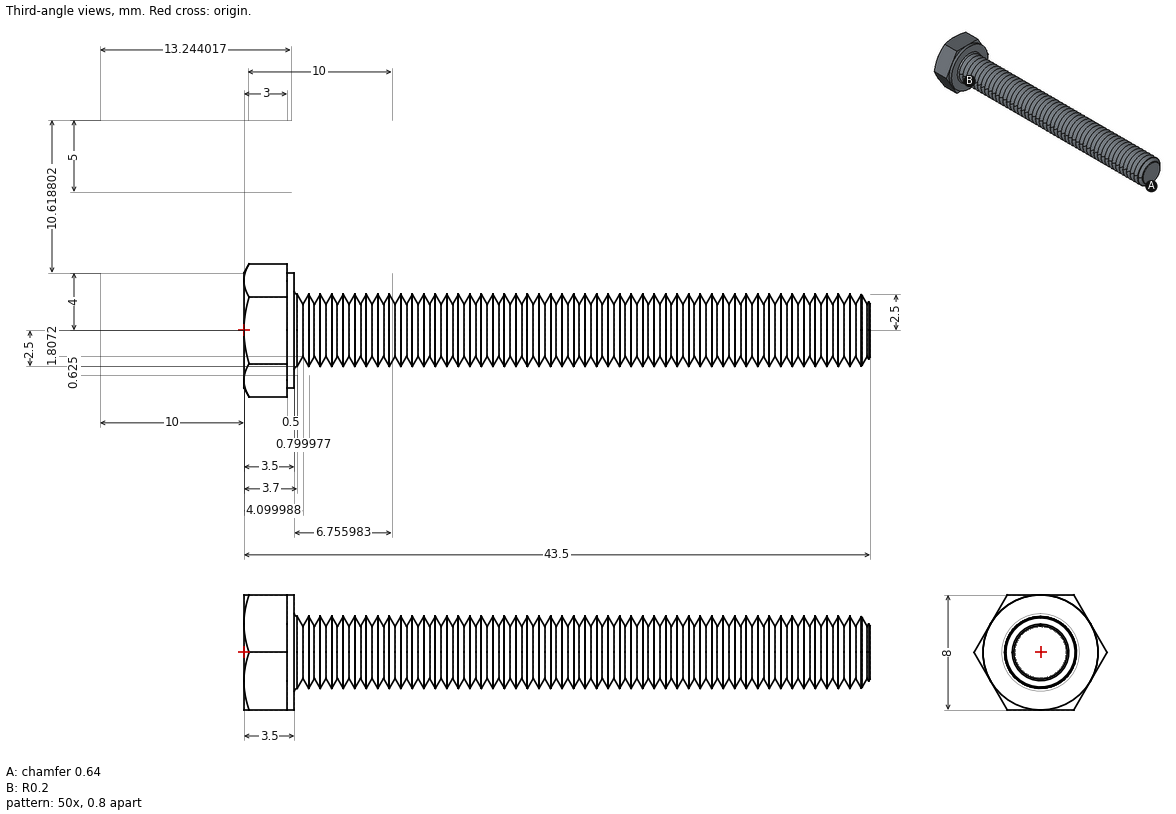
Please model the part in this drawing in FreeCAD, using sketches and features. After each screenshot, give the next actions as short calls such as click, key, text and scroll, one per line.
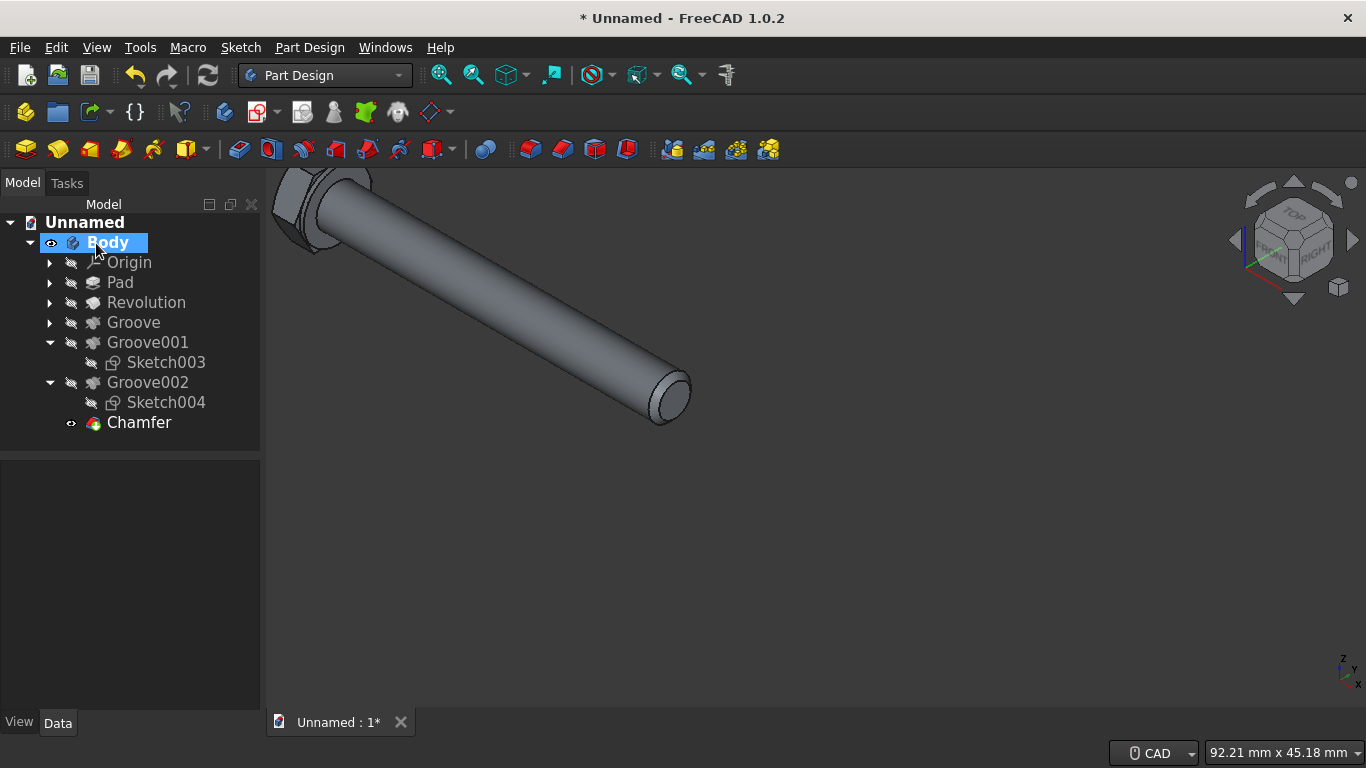
click(442, 76)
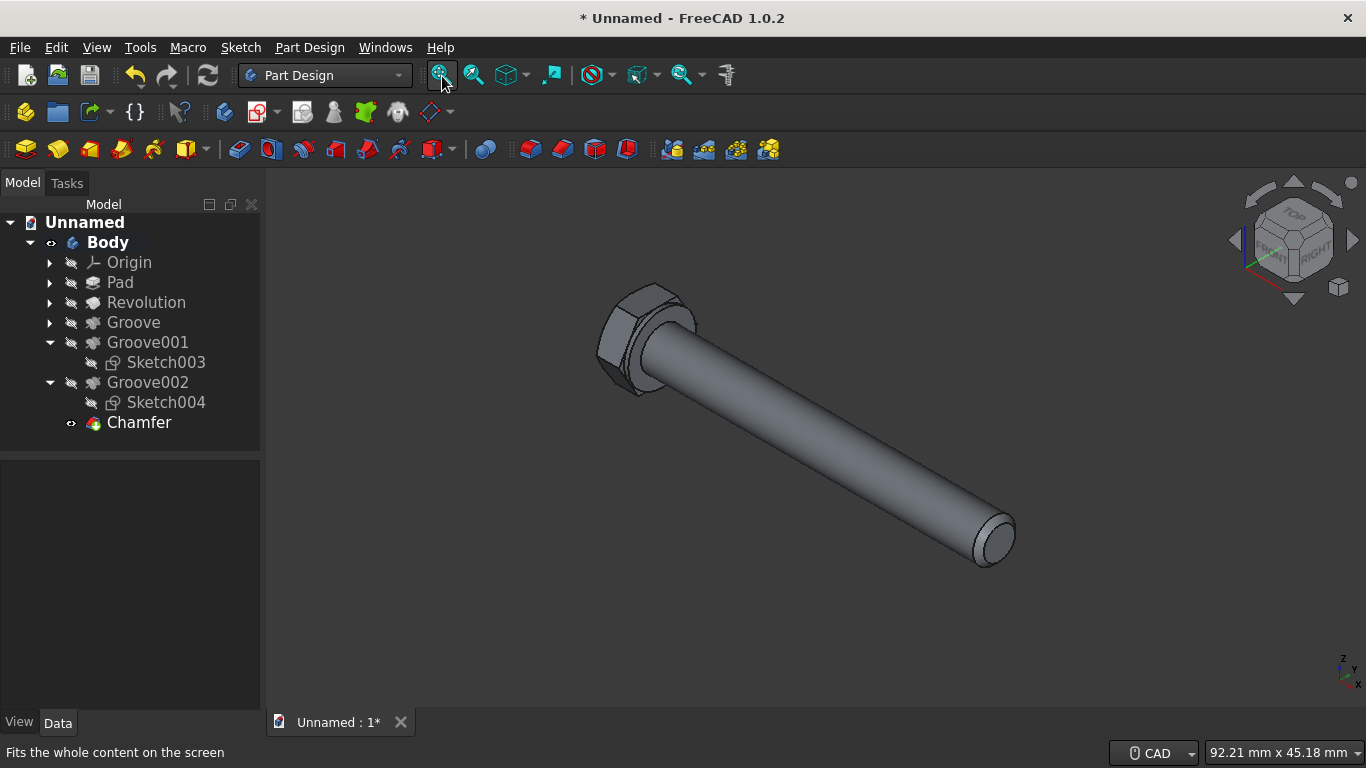
key(2)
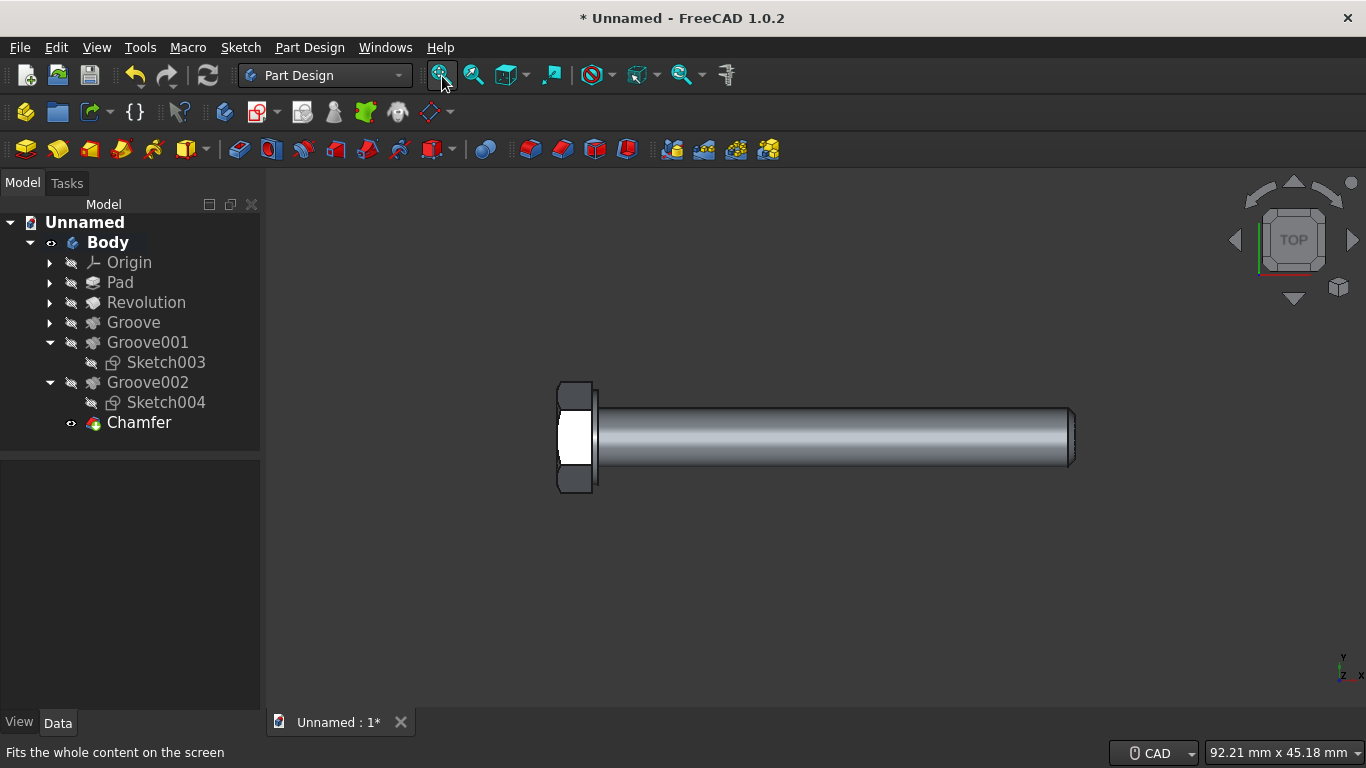
key(1)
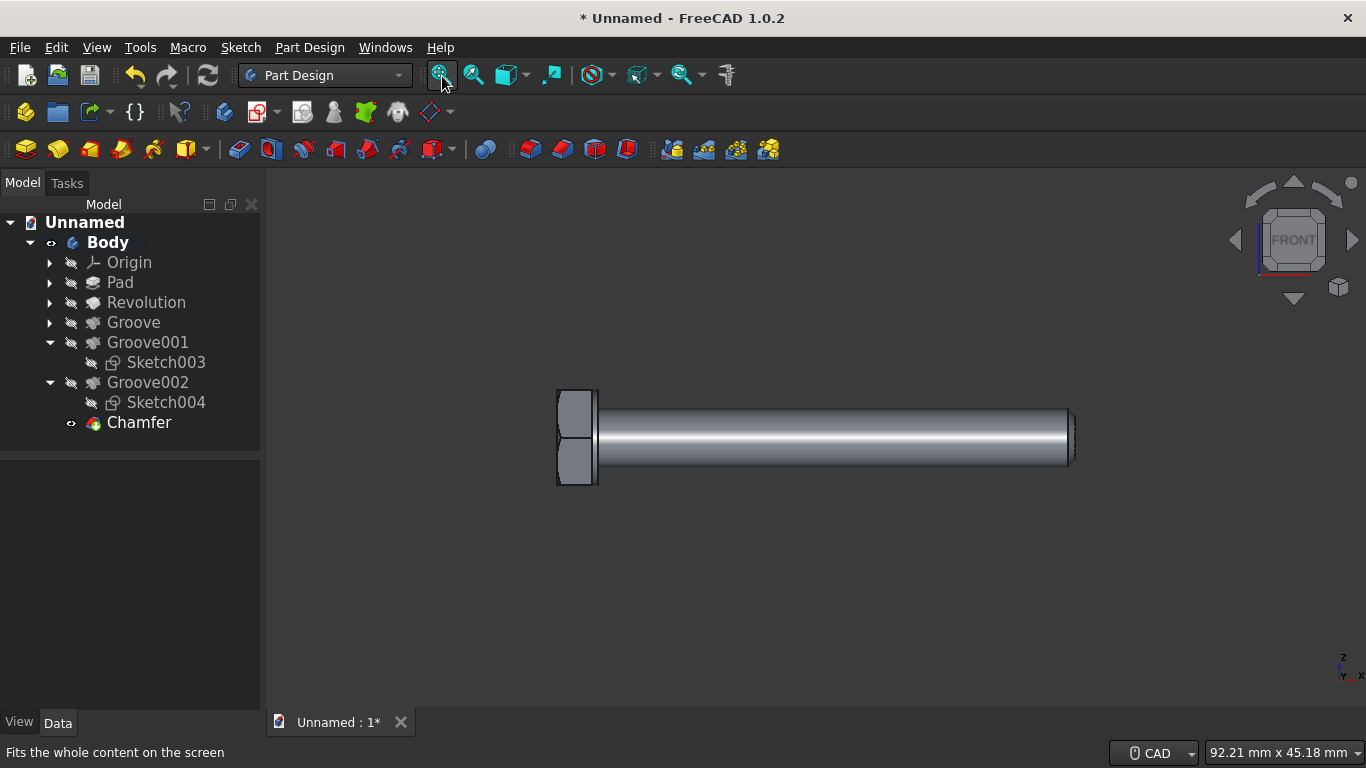
key(3)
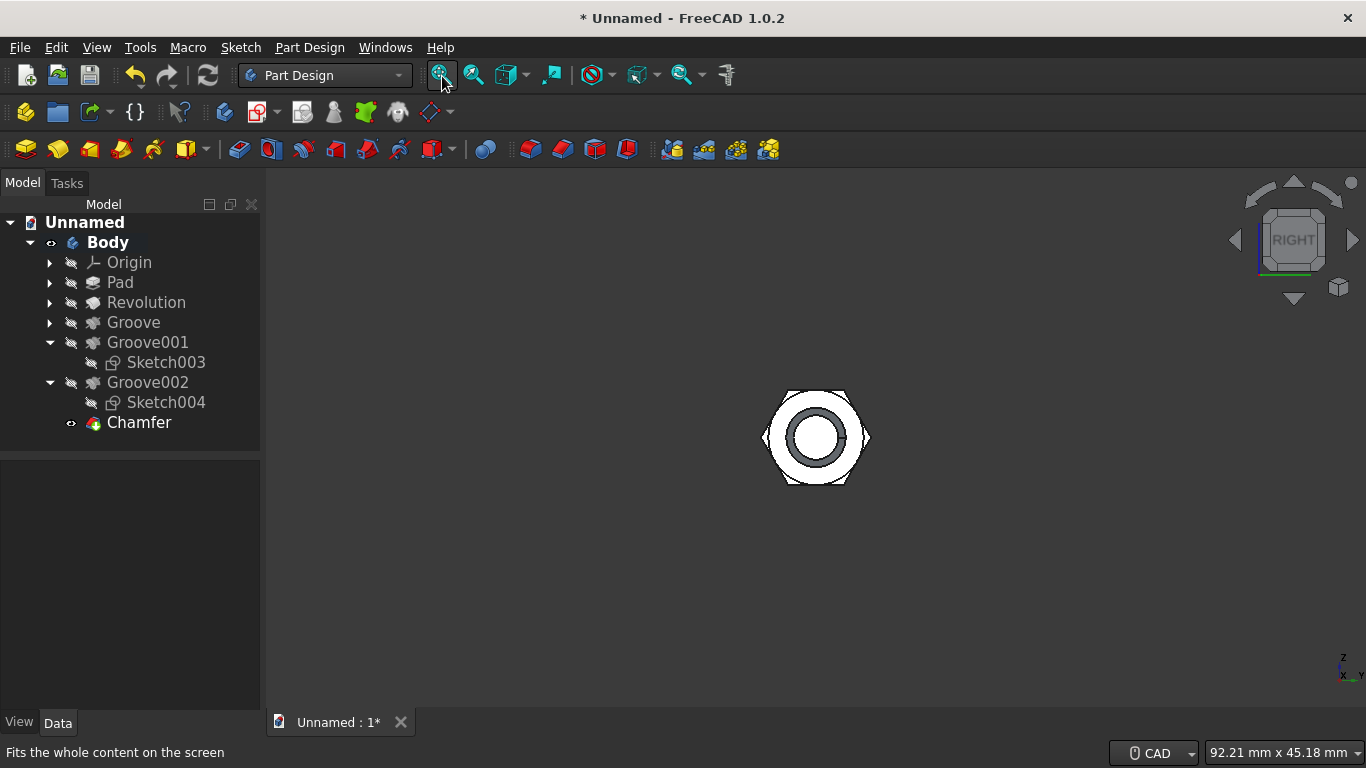
click(442, 76)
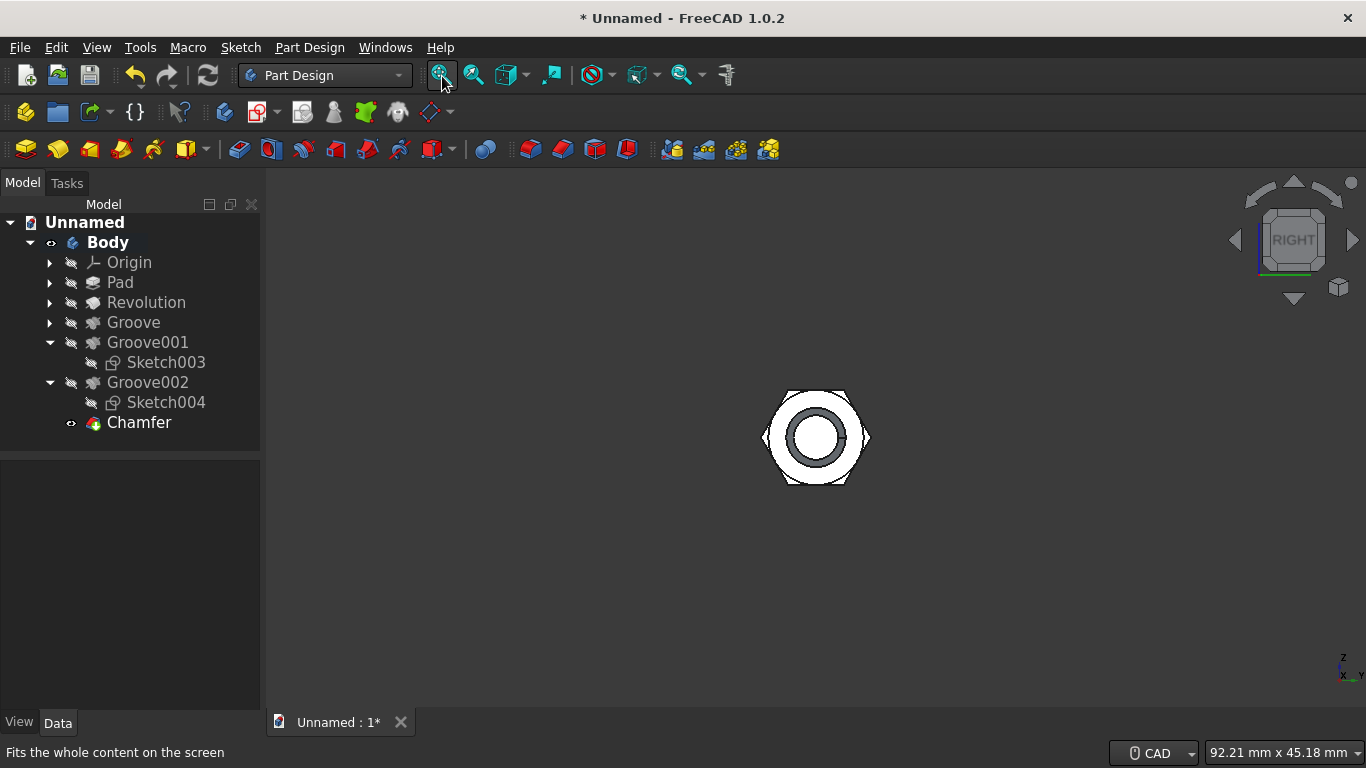
key(5)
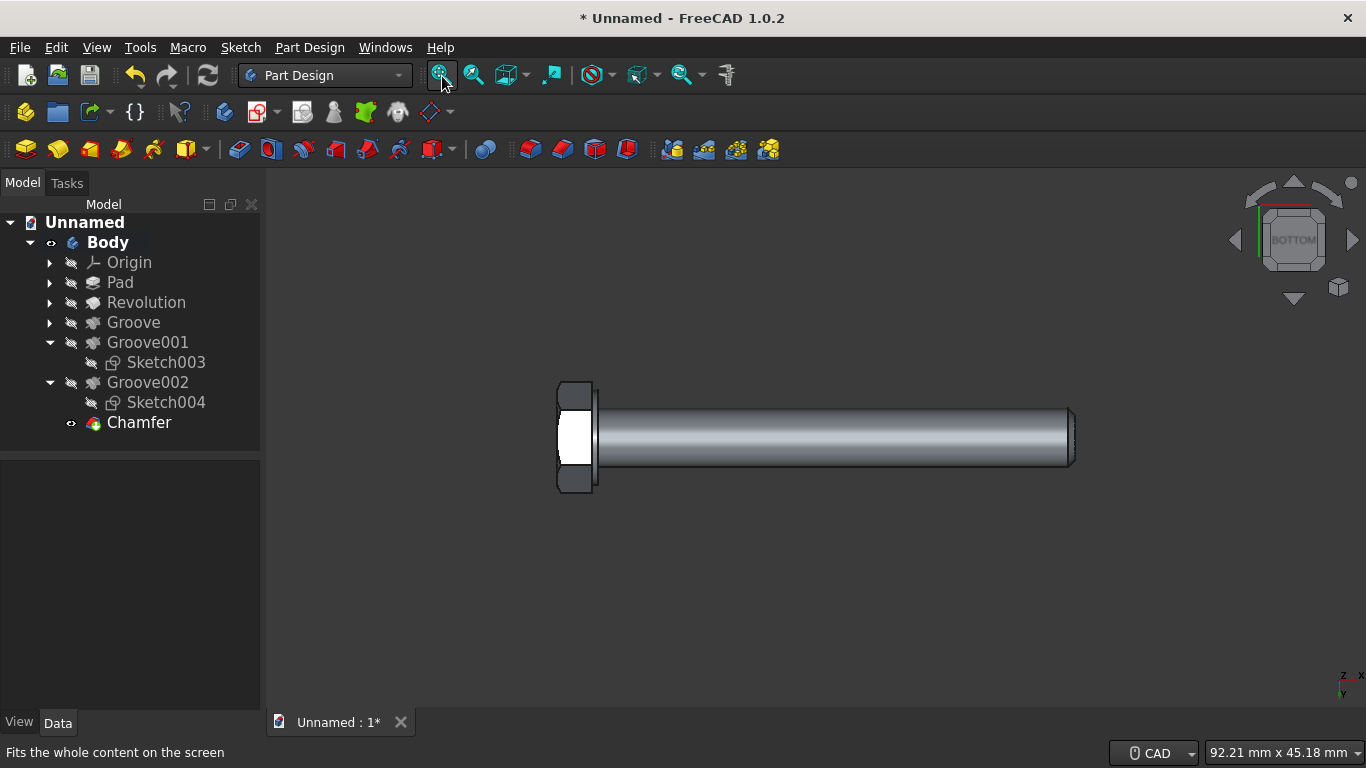
key(4)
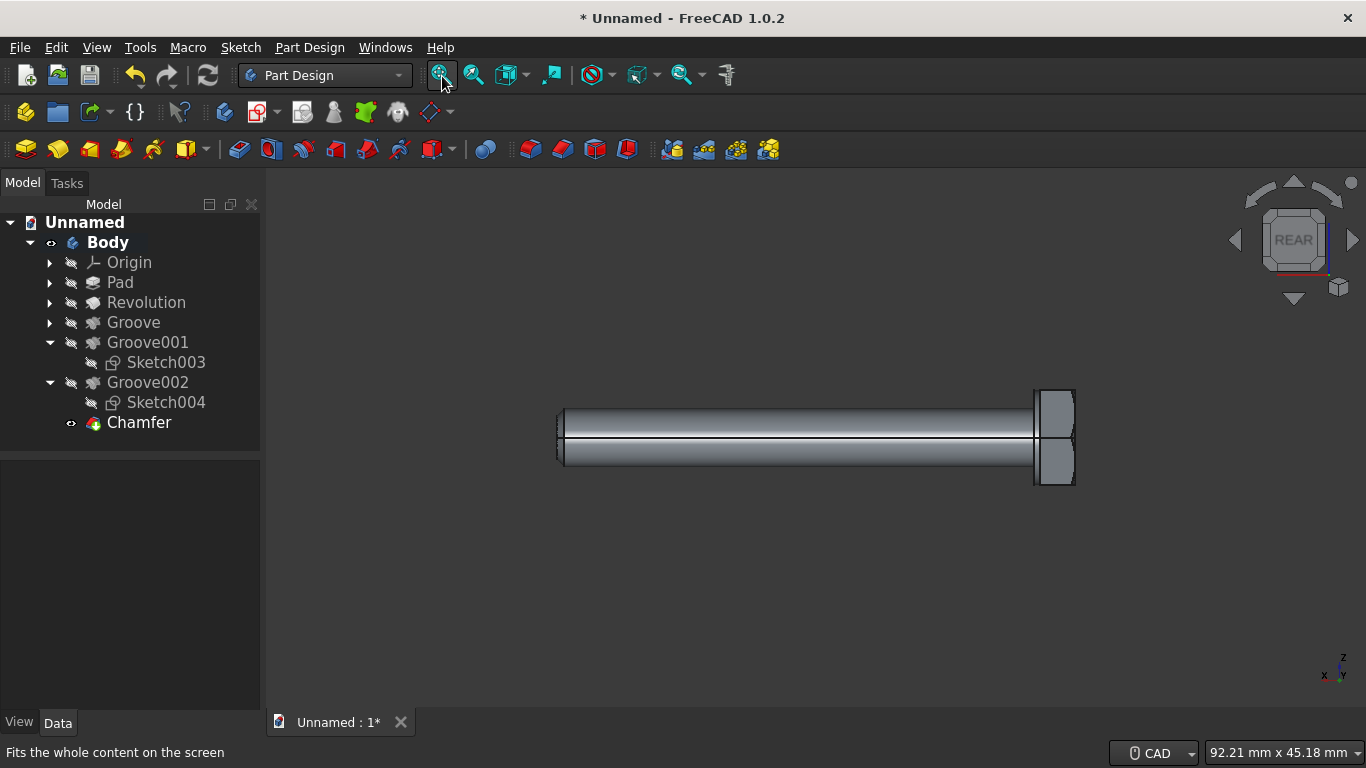
key(6)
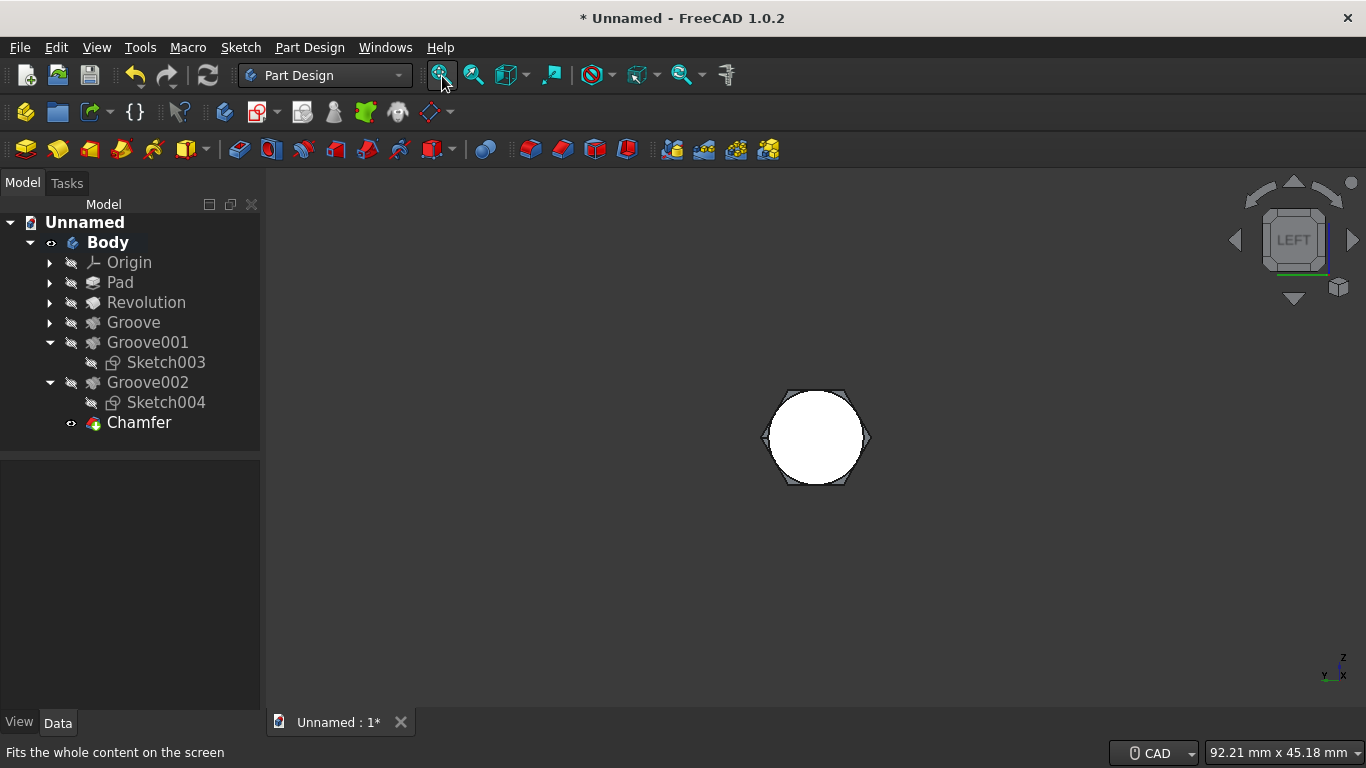
click(442, 76)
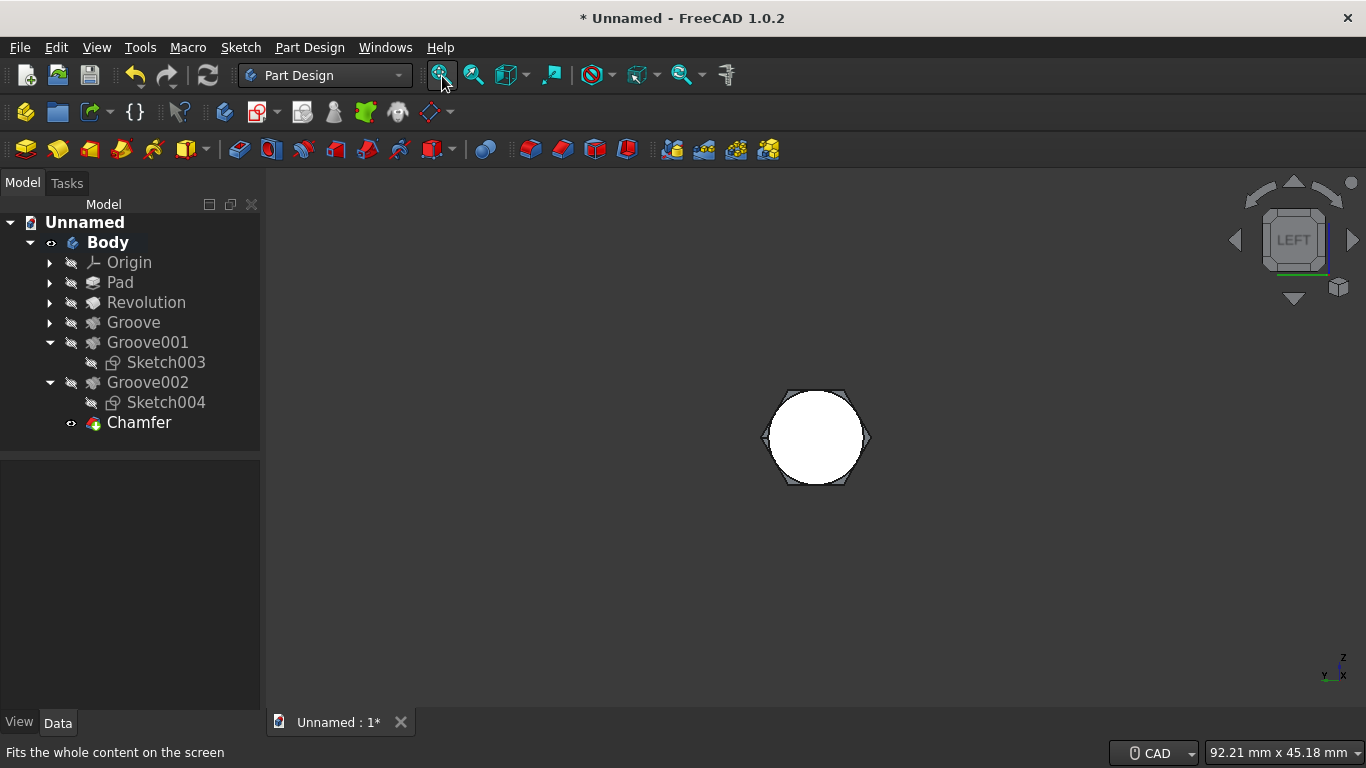
key(v)
key(3)